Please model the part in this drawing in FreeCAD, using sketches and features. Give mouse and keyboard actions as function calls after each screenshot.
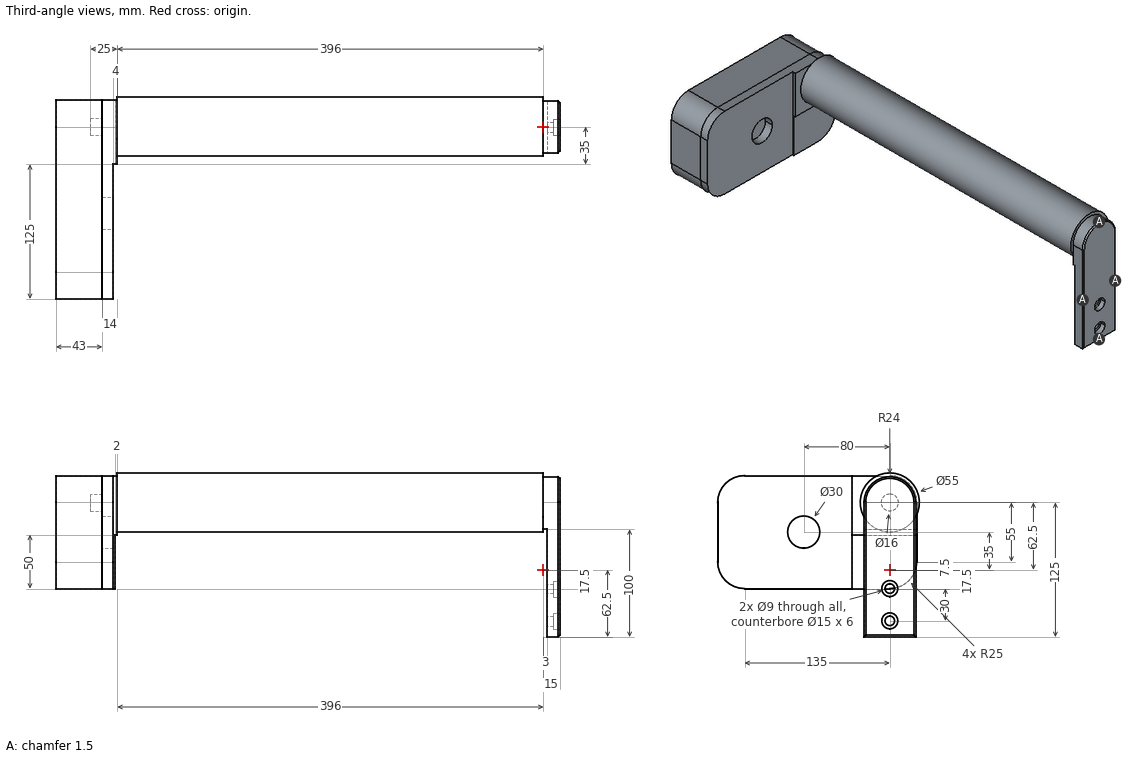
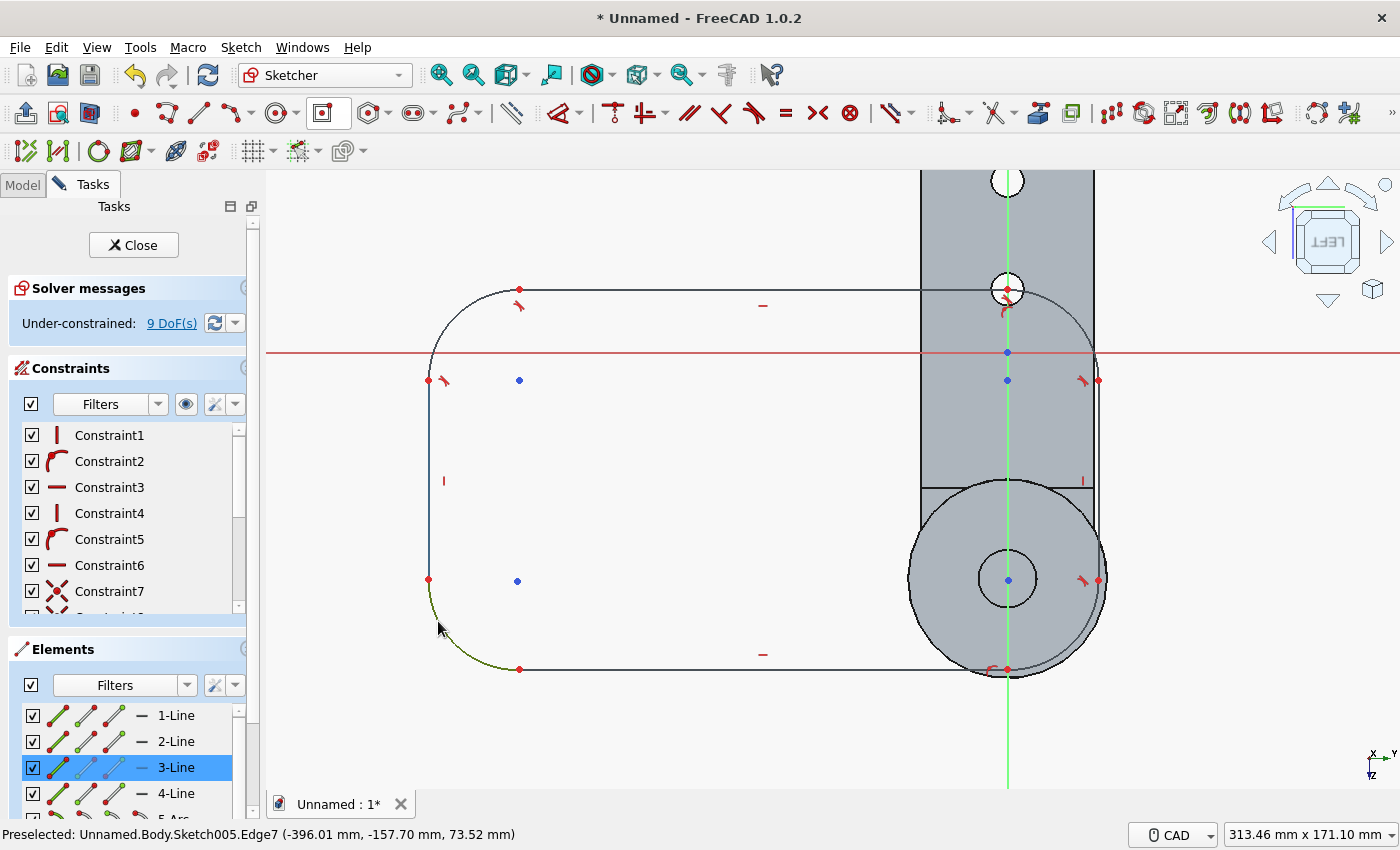
key(t)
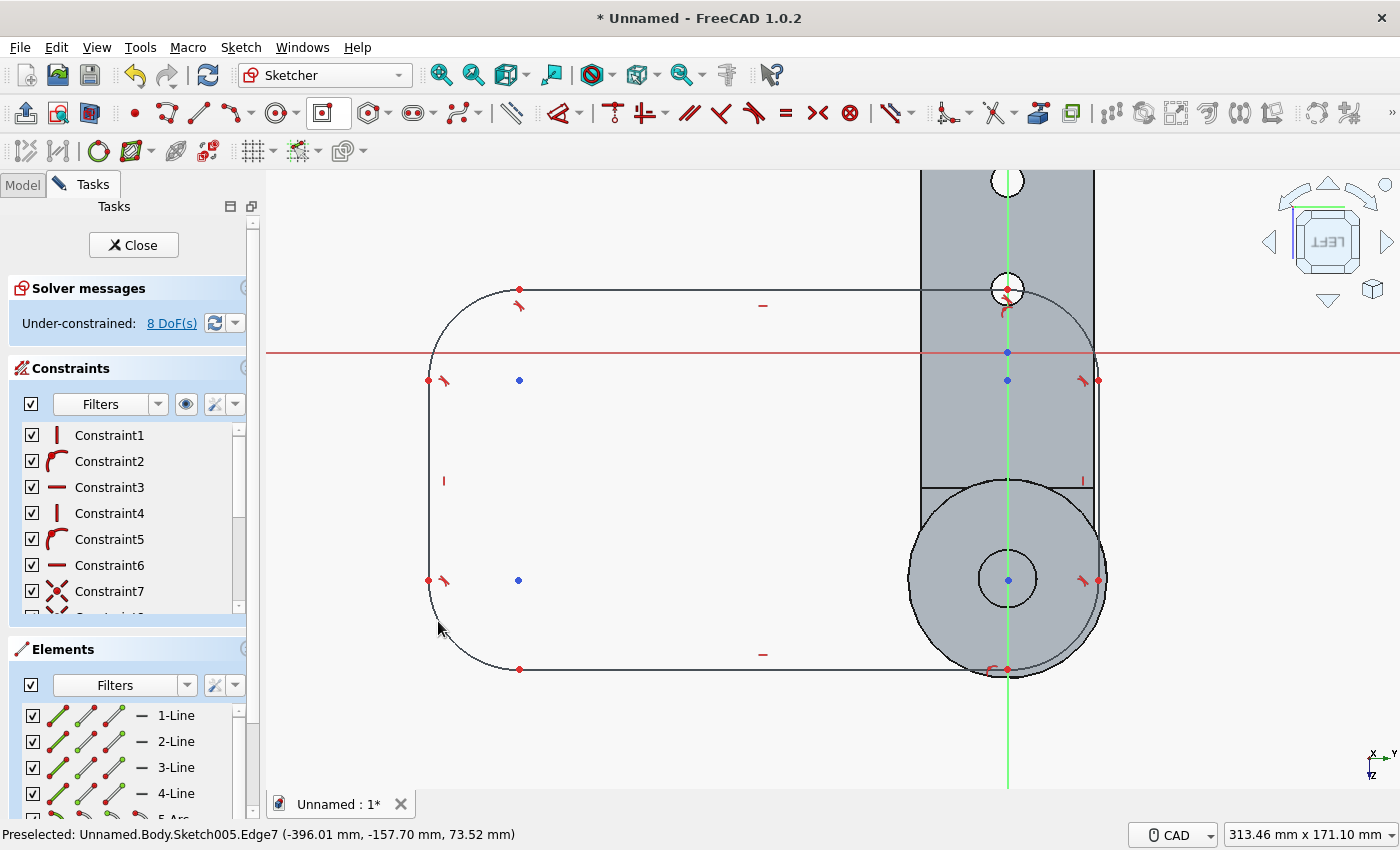
click(666, 670)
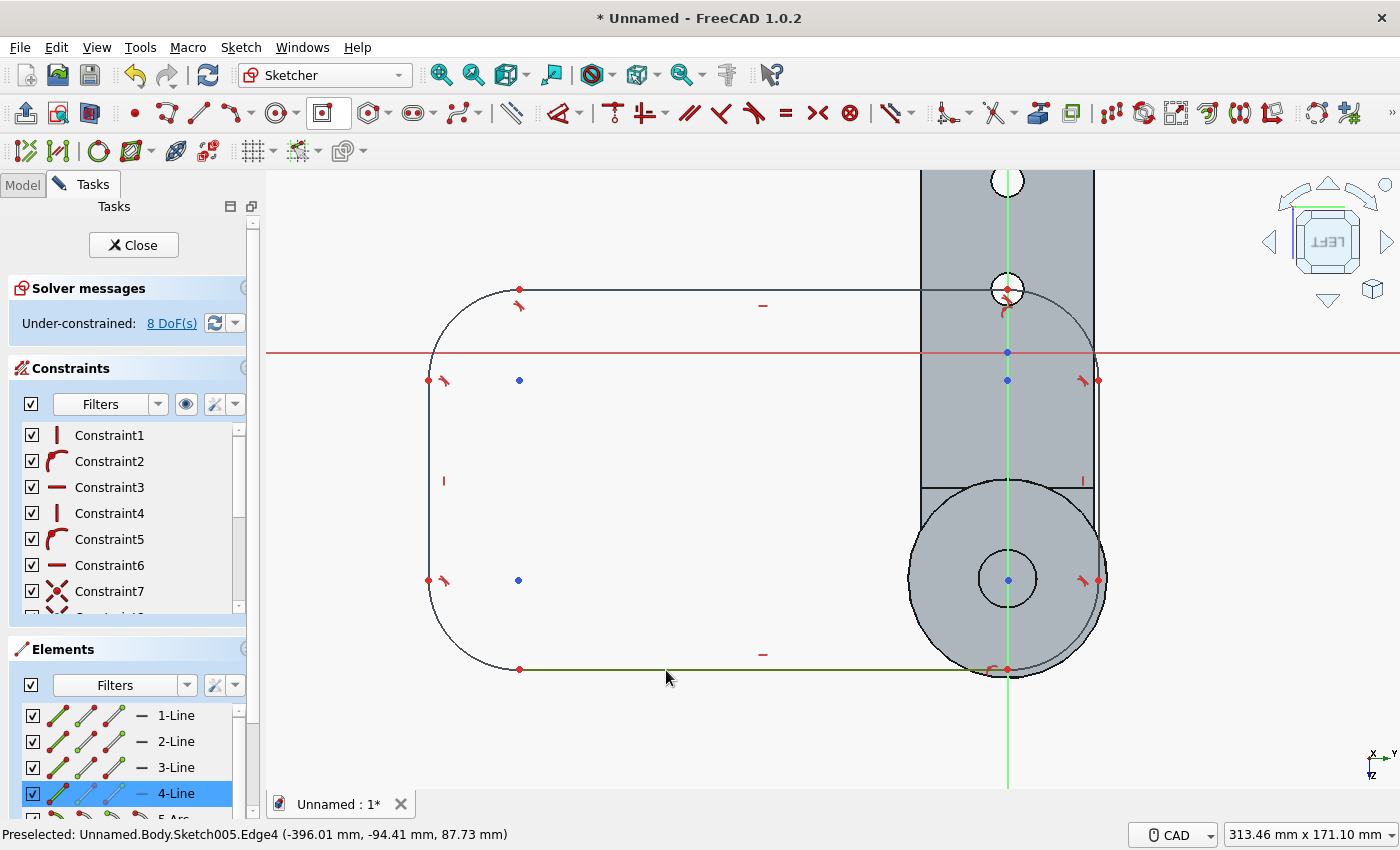
click(439, 621)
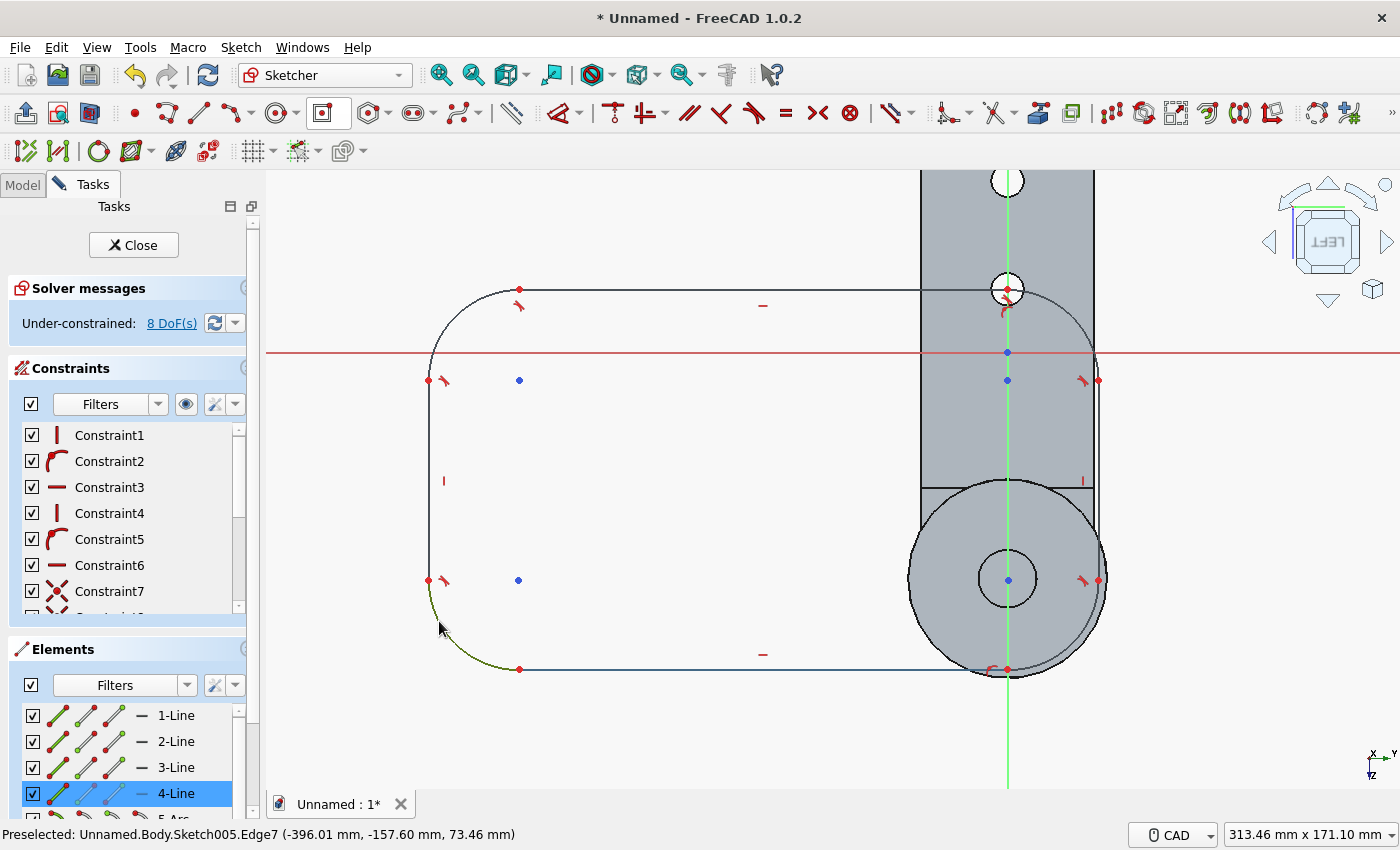
key(t)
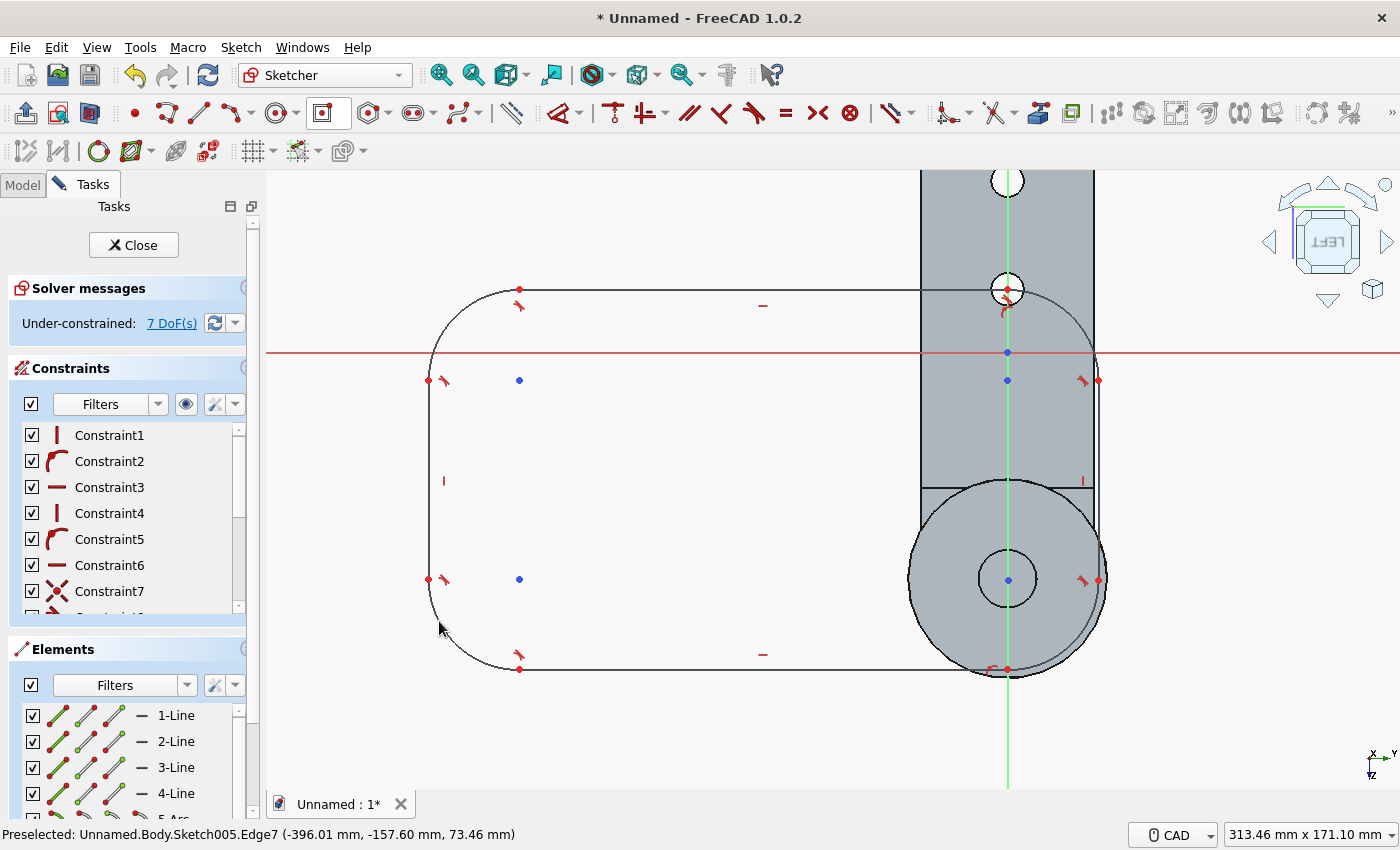
click(666, 670)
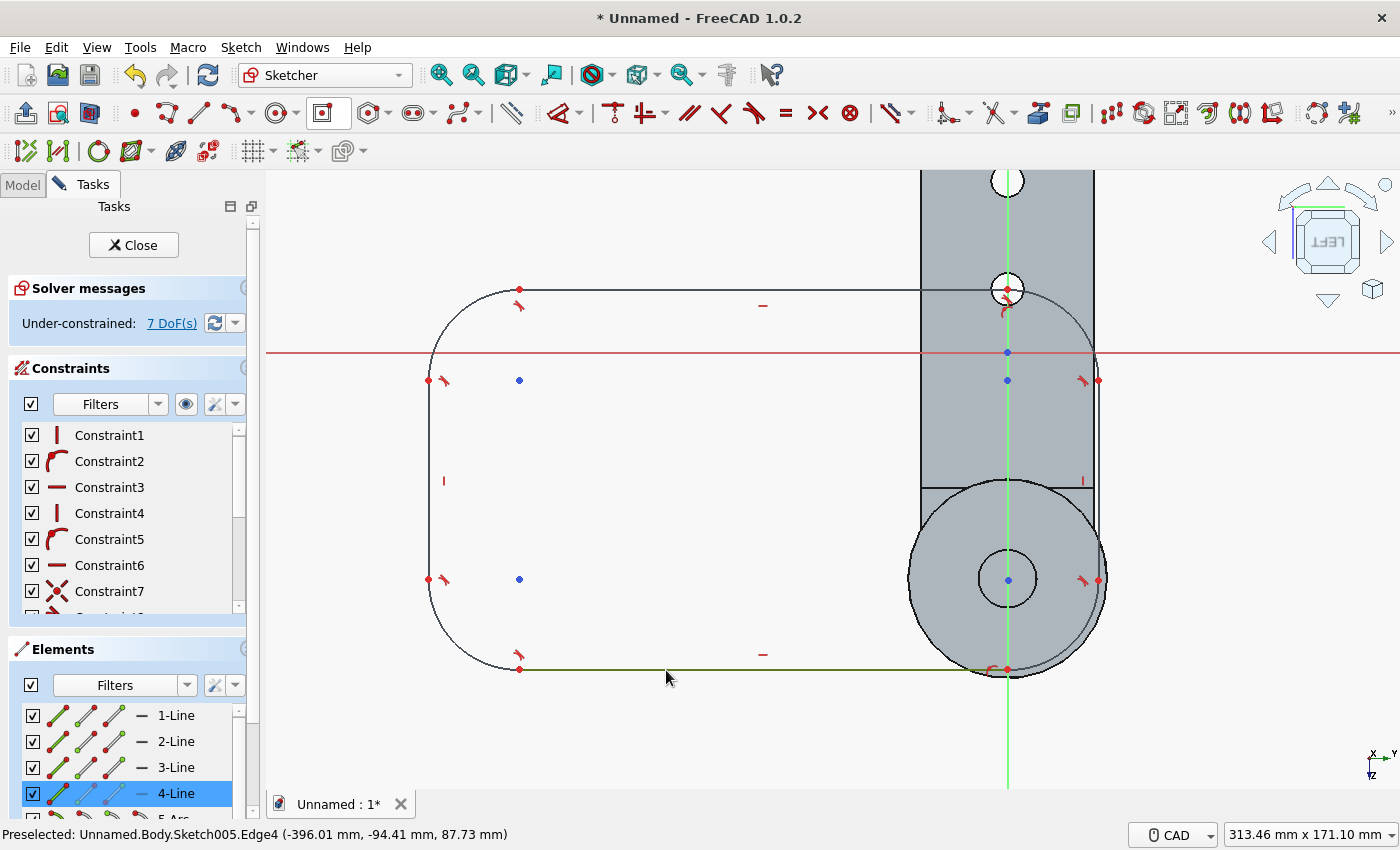
click(1049, 661)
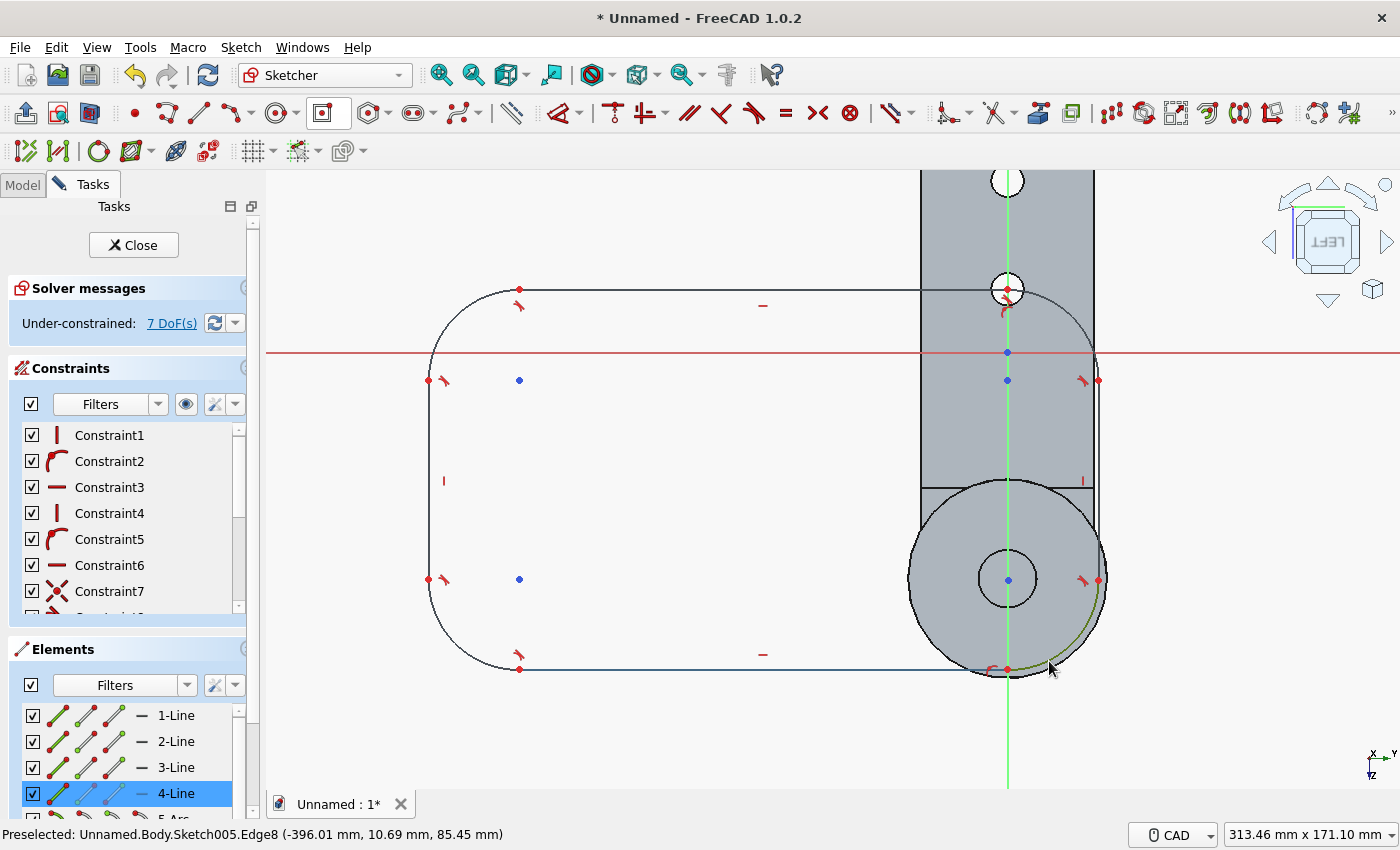
key(t)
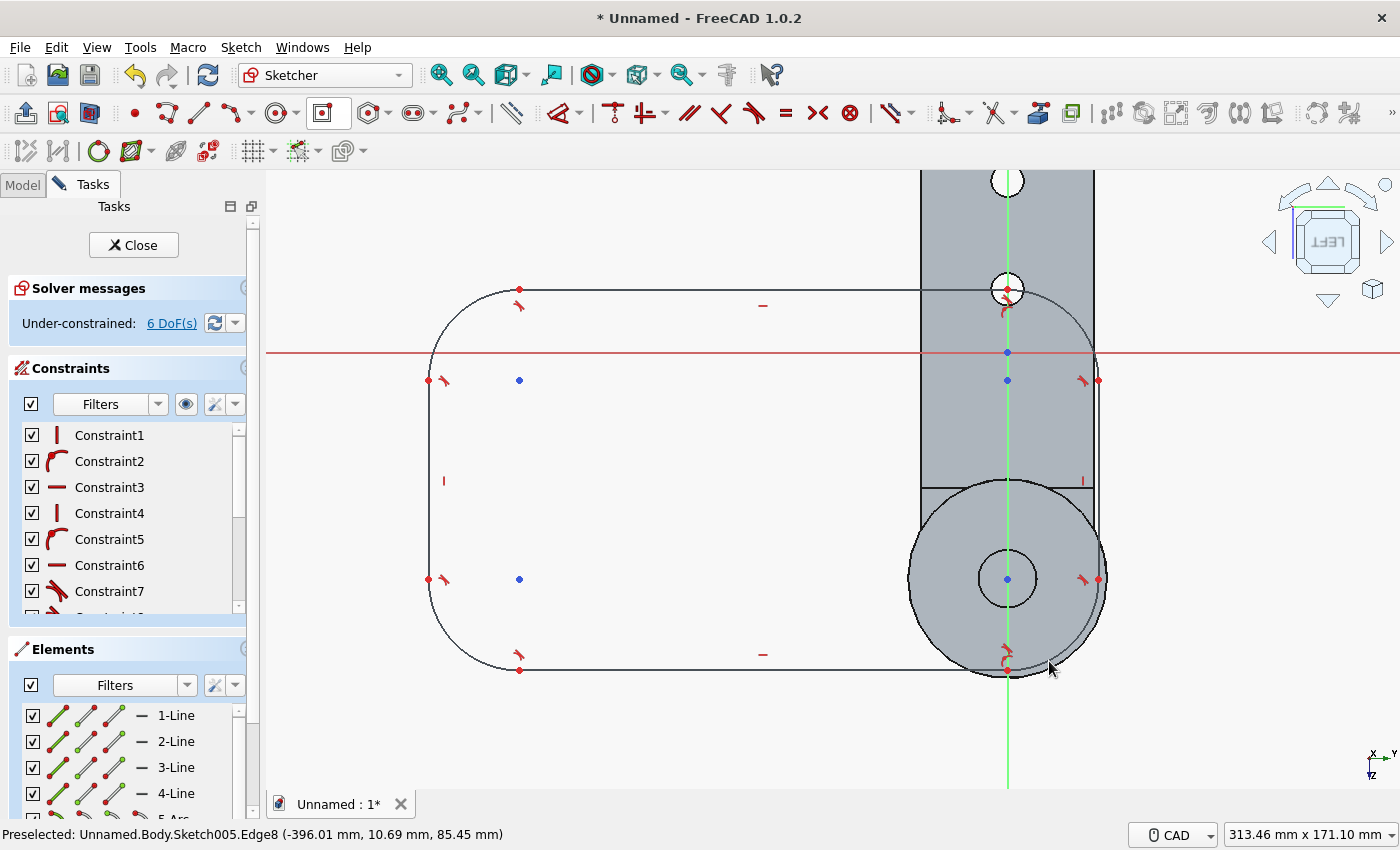
click(1089, 340)